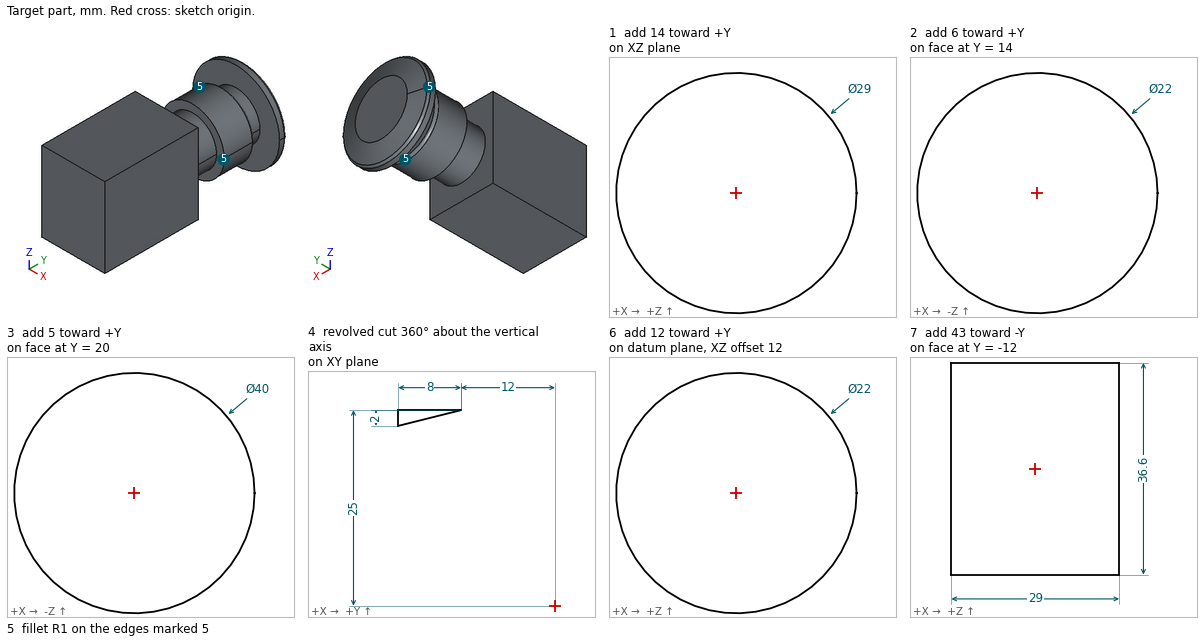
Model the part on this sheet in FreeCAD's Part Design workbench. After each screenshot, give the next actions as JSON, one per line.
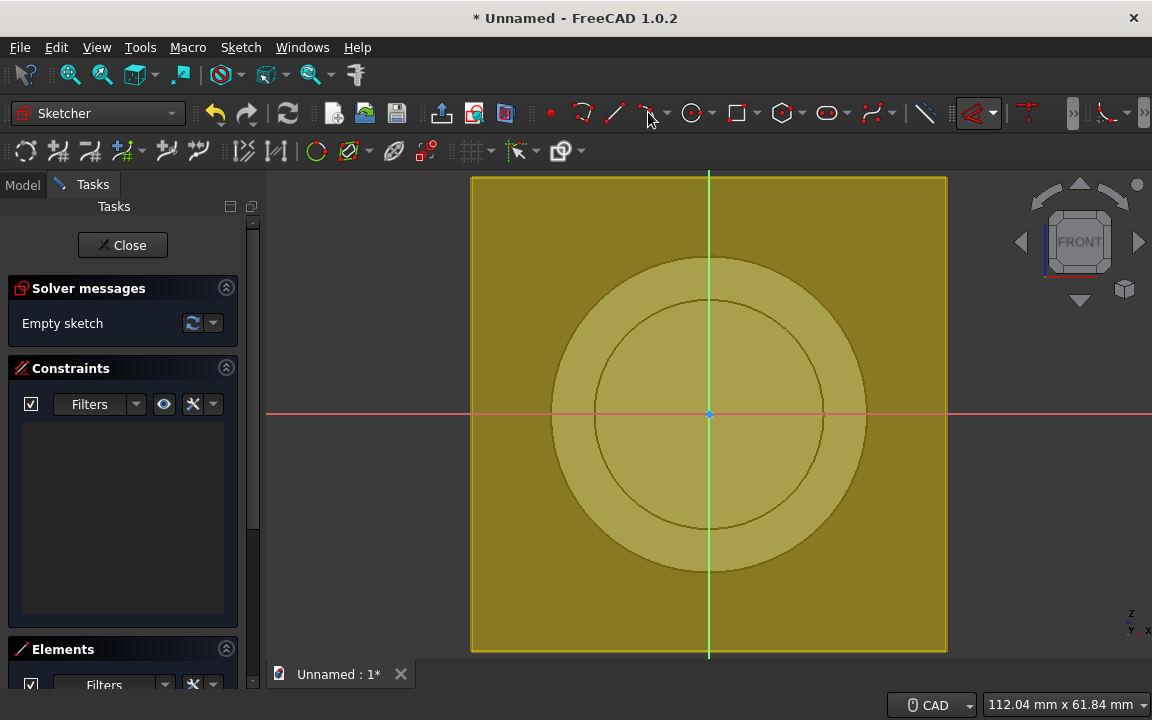
{"action": "scroll", "coordinate": [792, 414], "scroll_direction": "up", "scroll_amount": 3}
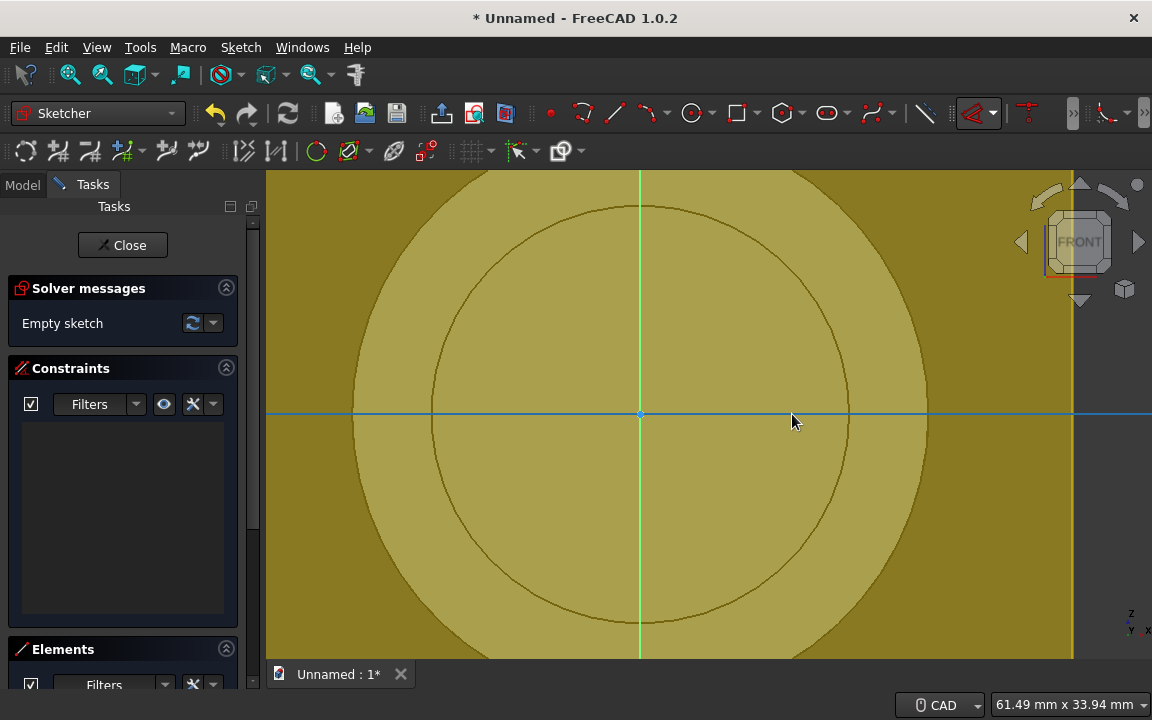
{"action": "left_click", "coordinate": [692, 114]}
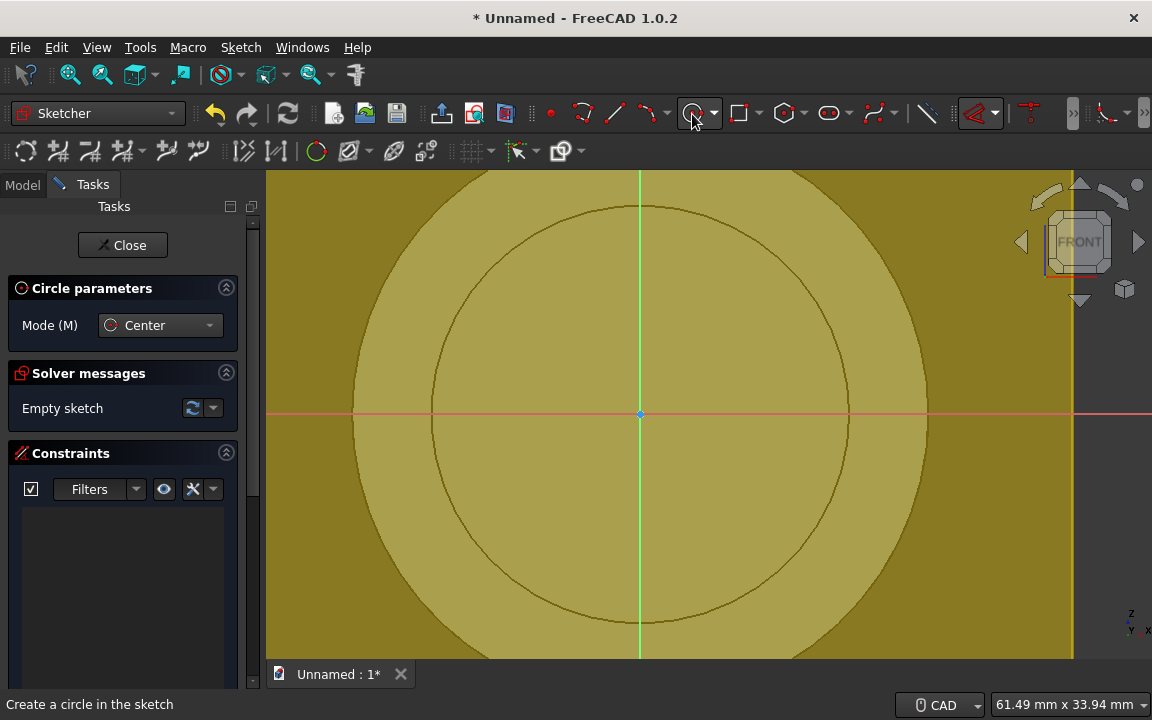
{"action": "left_click", "coordinate": [640, 414]}
{"action": "left_click", "coordinate": [752, 302]}
{"action": "key", "text": "Escape"}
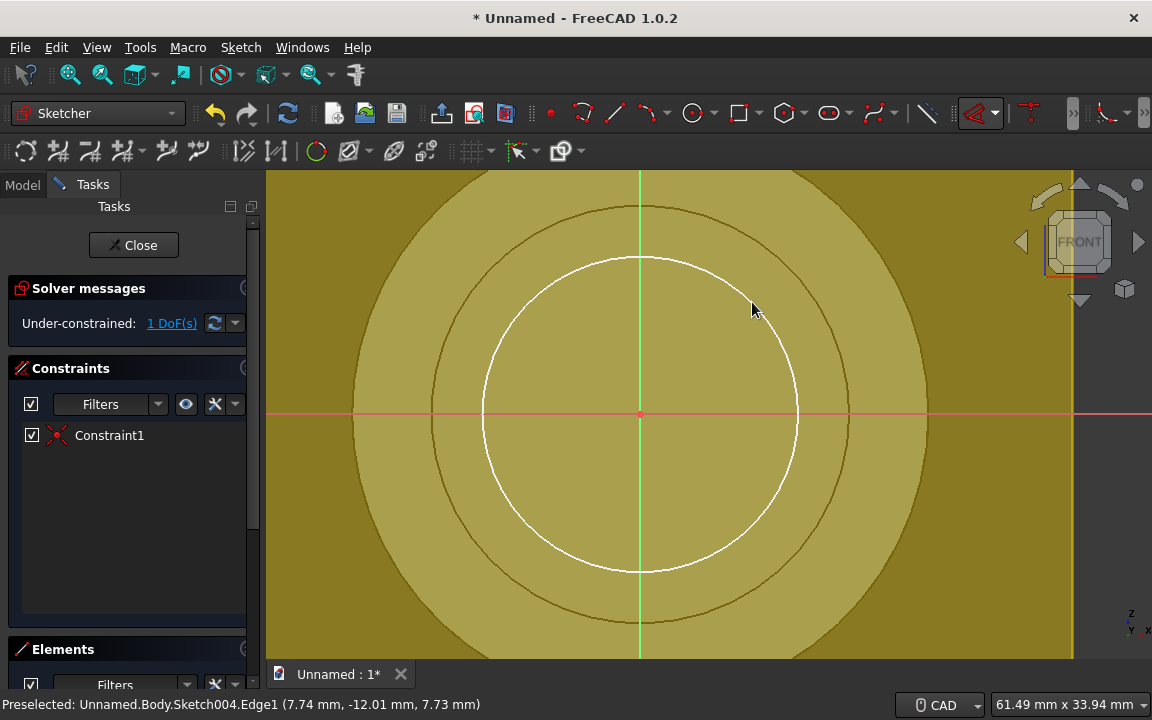
{"action": "left_click", "coordinate": [752, 303]}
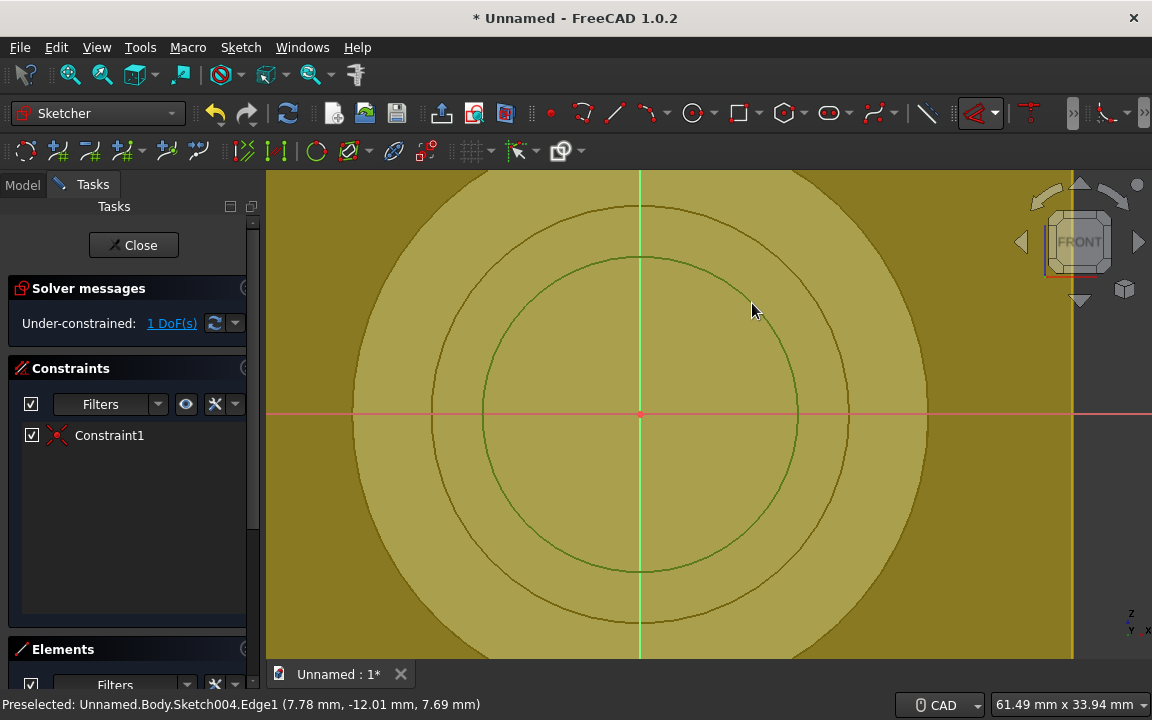
{"action": "key", "text": "k o"}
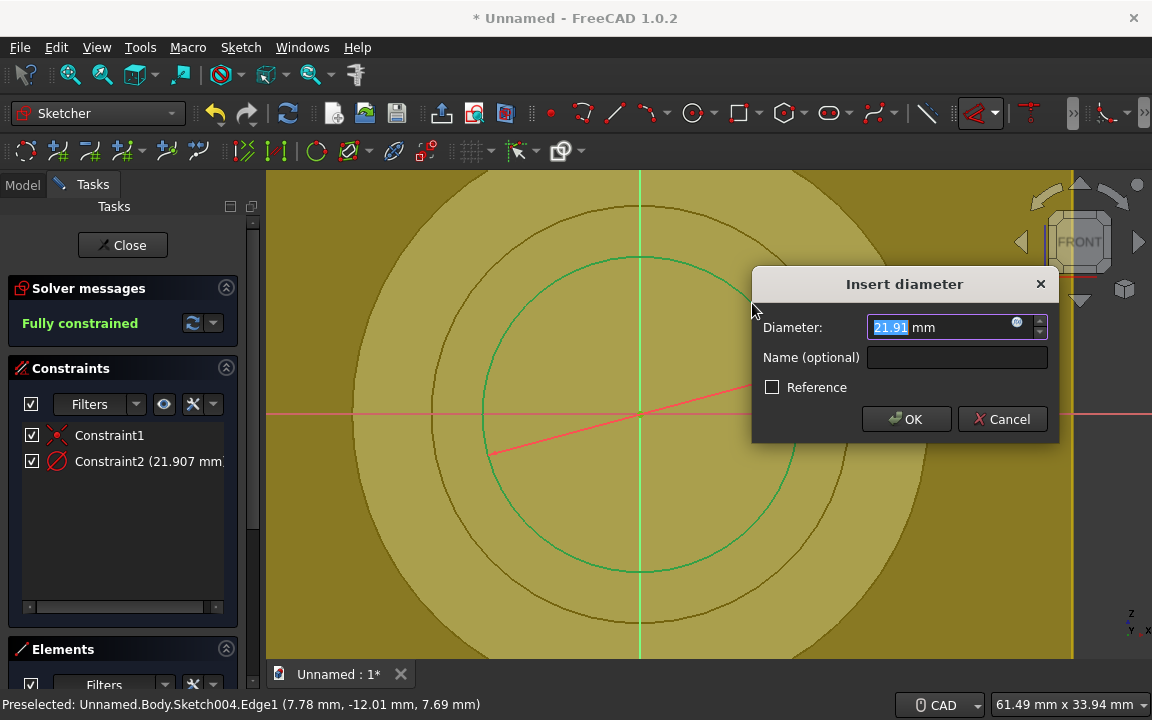
{"action": "type", "text": "22"}
{"action": "key", "text": "Return"}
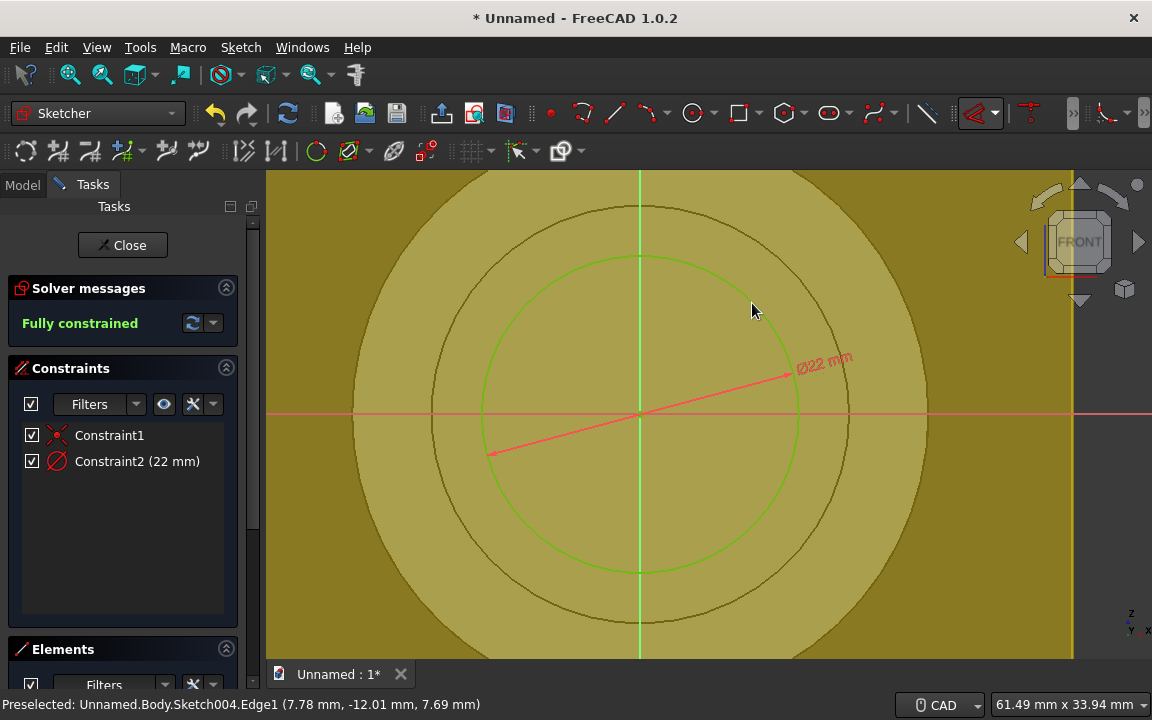
{"action": "left_click", "coordinate": [123, 245]}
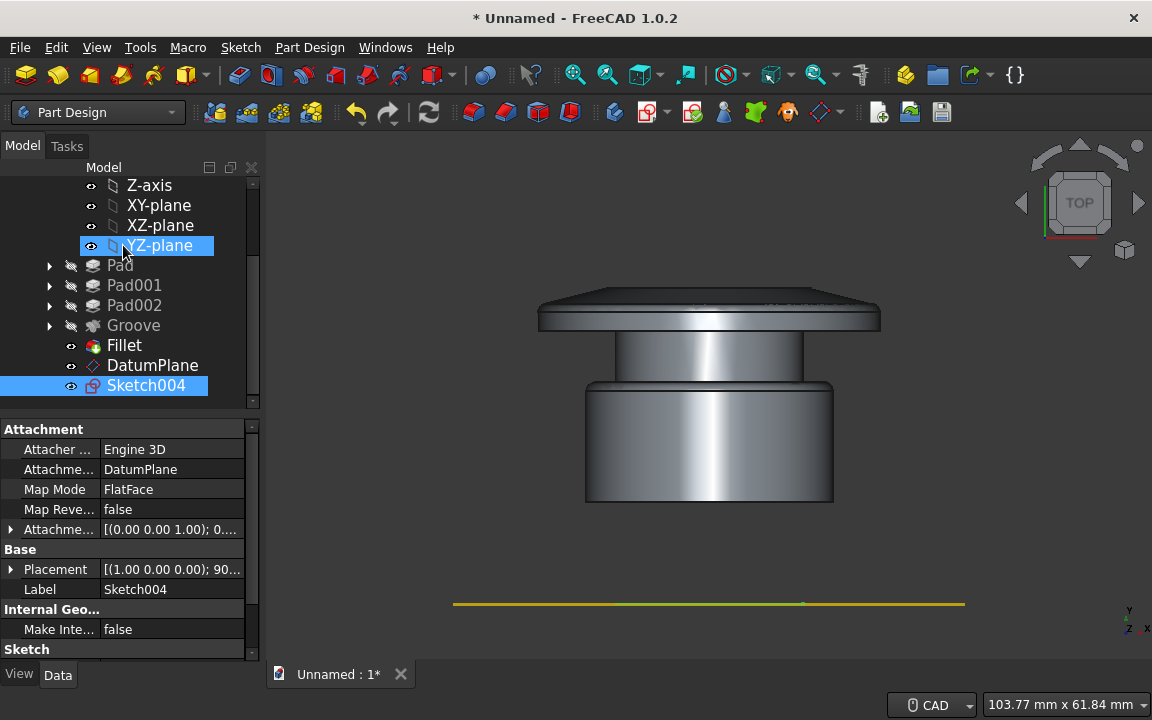
{"action": "left_click", "coordinate": [26, 76]}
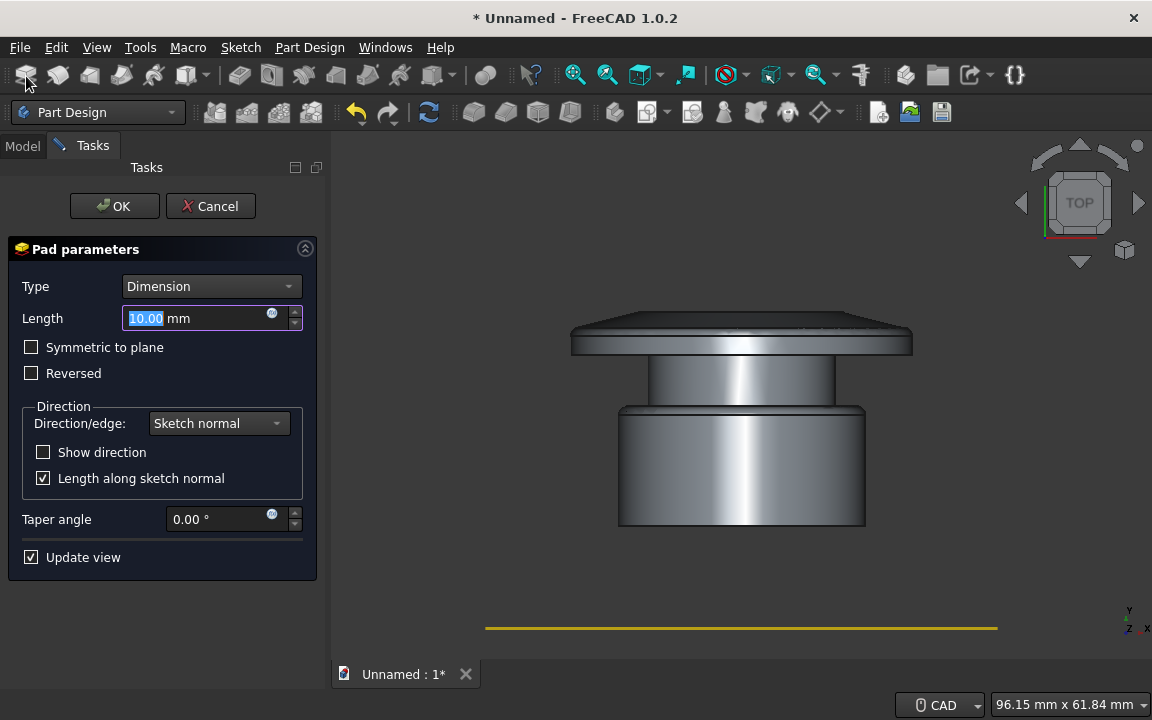
{"action": "type", "text": "12"}
{"action": "key", "text": "Tab"}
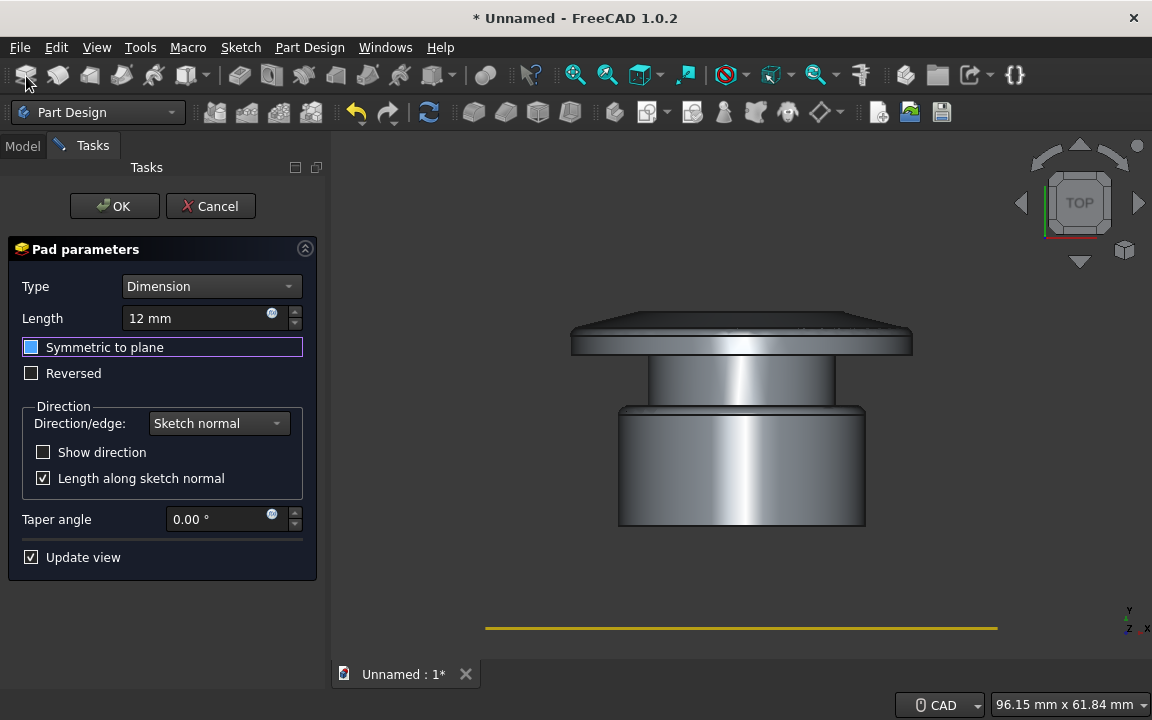
{"action": "left_click", "coordinate": [30, 373]}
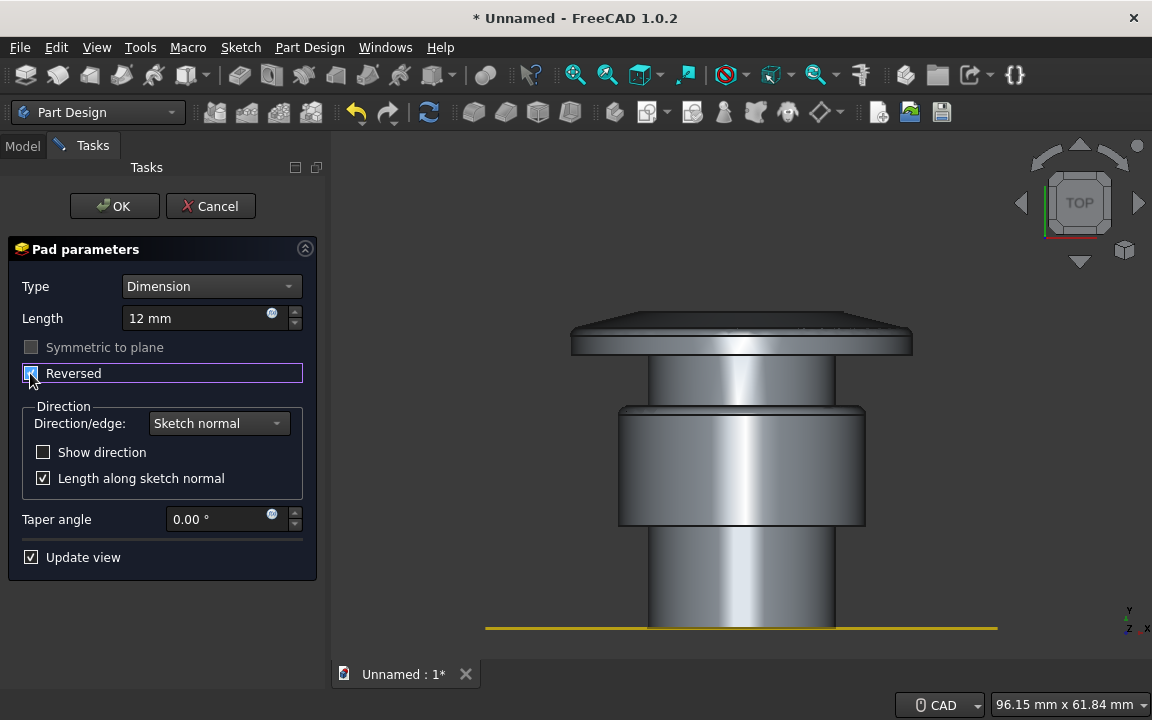
{"action": "left_click", "coordinate": [115, 206]}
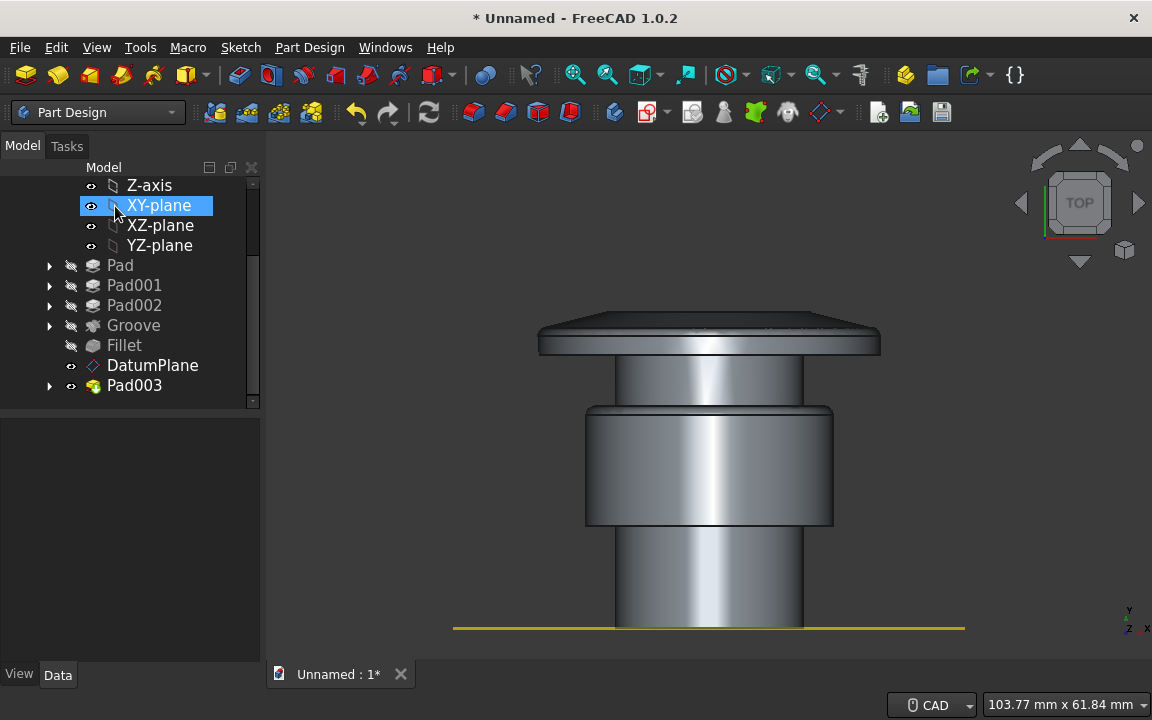
{"action": "left_click", "coordinate": [116, 366]}
{"action": "key", "text": "space"}